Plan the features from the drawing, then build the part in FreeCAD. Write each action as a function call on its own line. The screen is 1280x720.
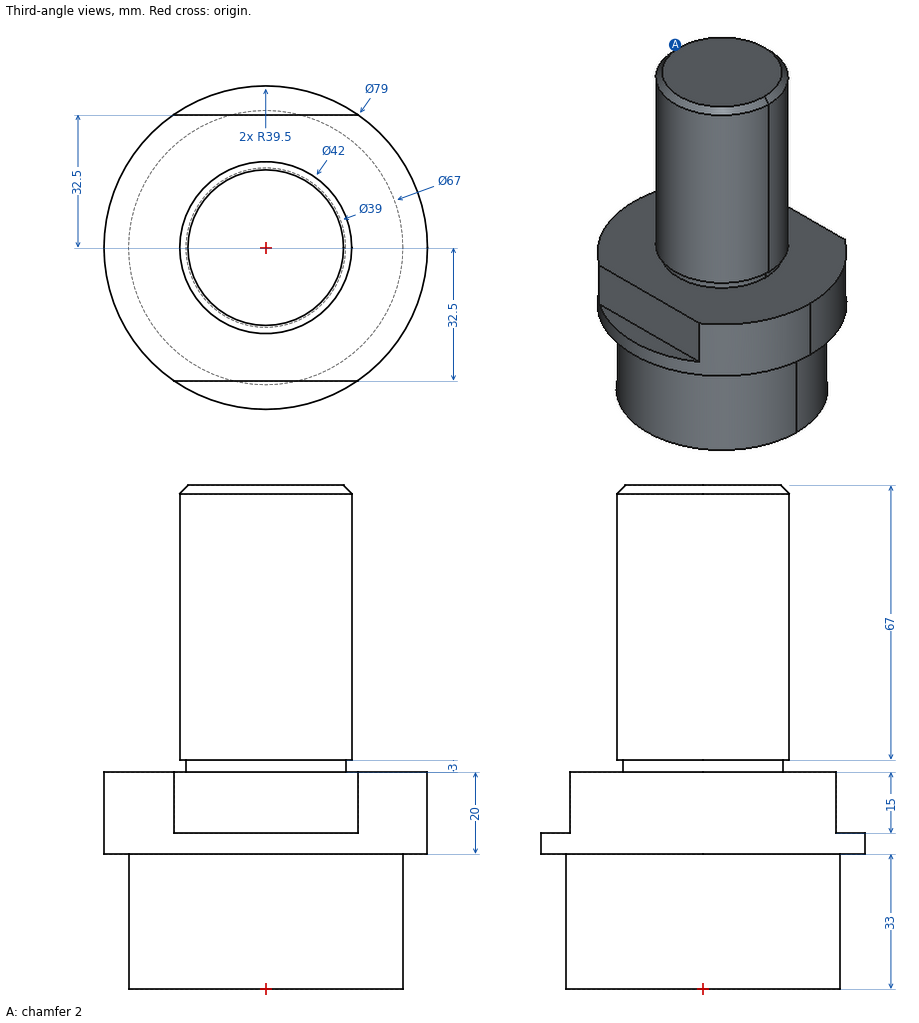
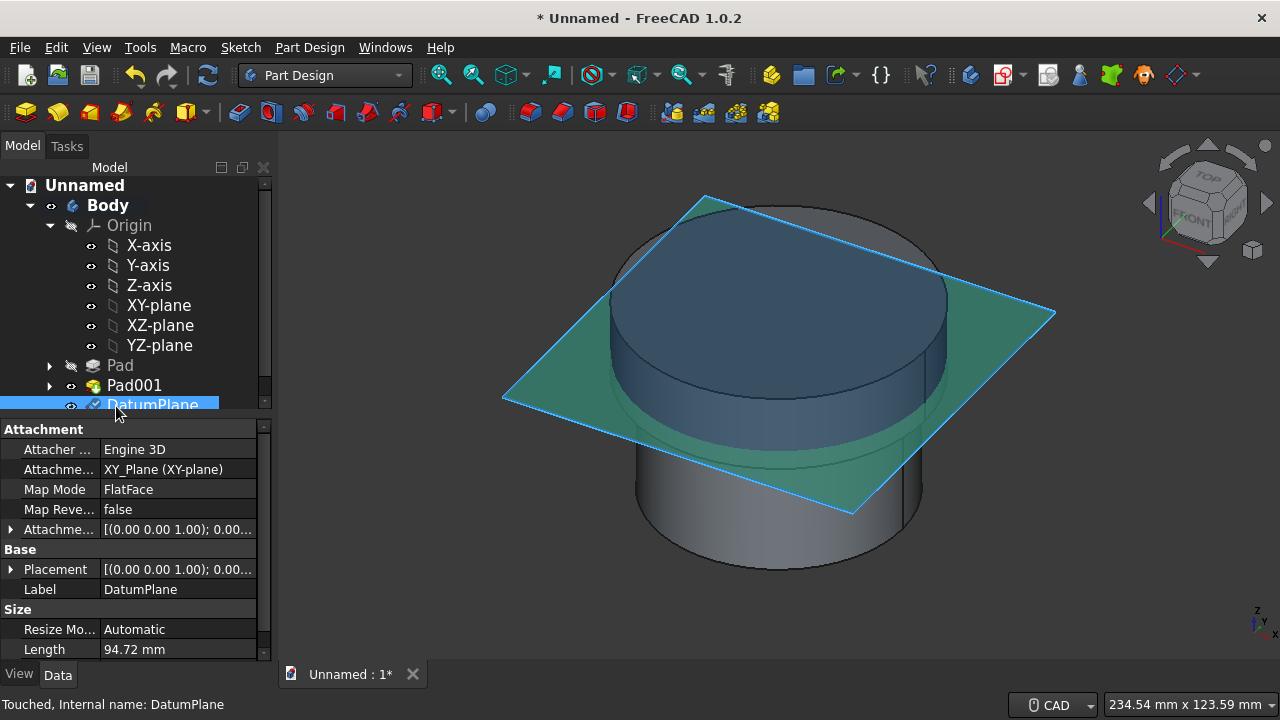
click(1004, 76)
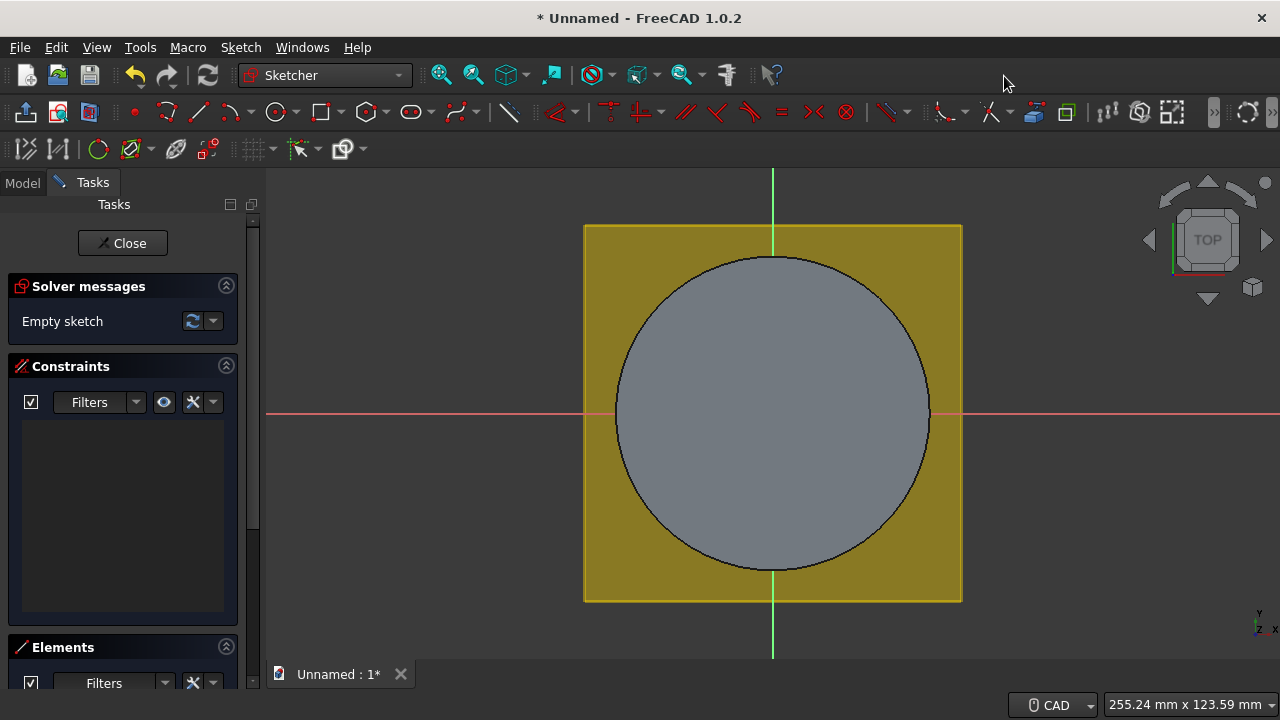
click(90, 112)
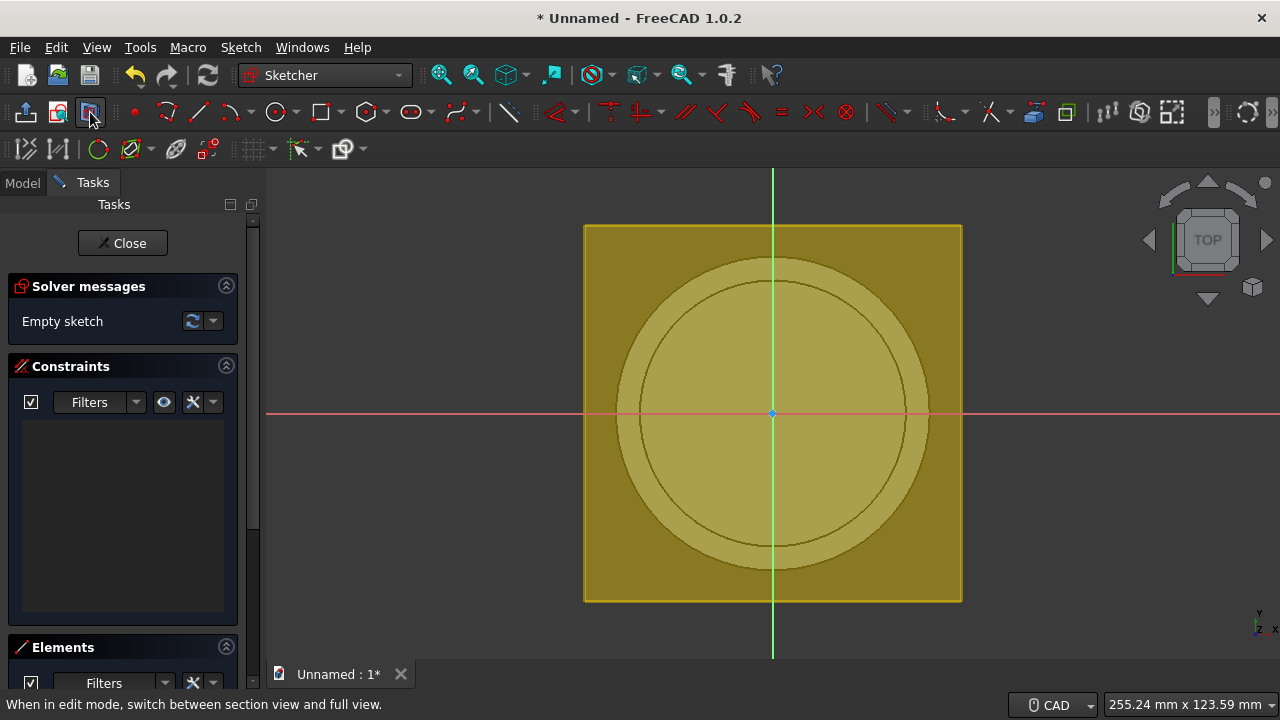
click(200, 112)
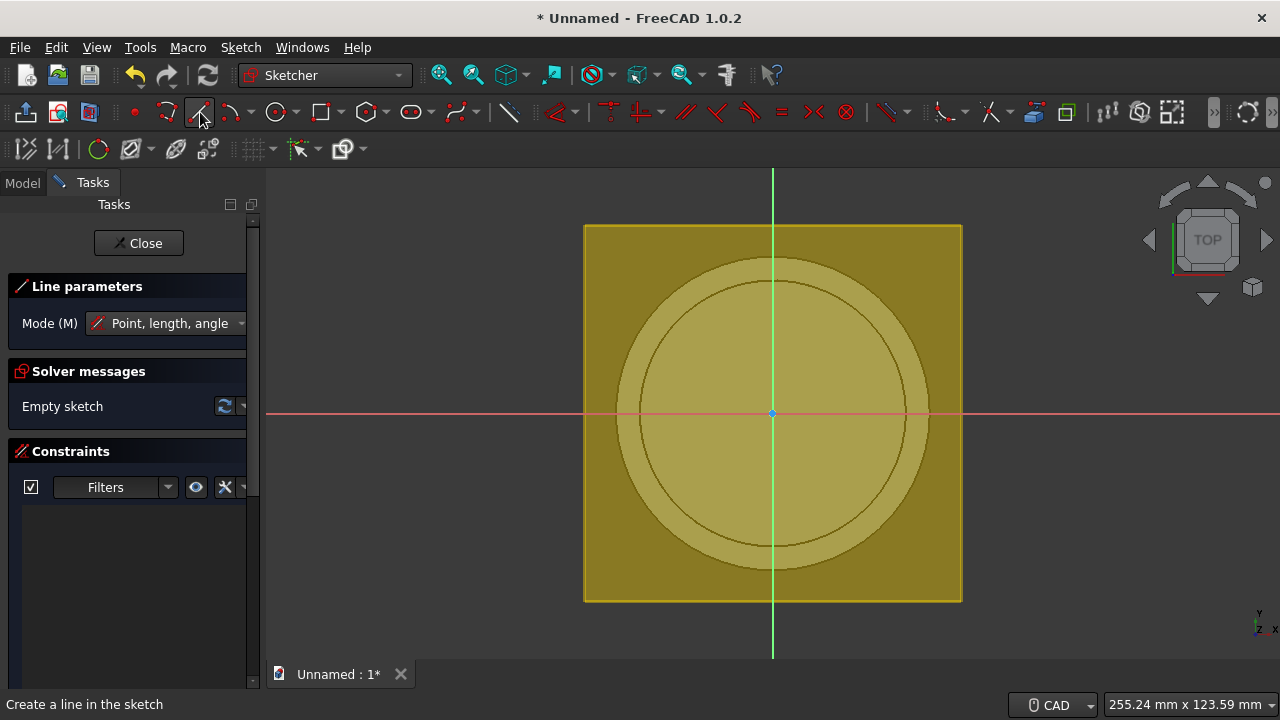
click(684, 284)
click(862, 284)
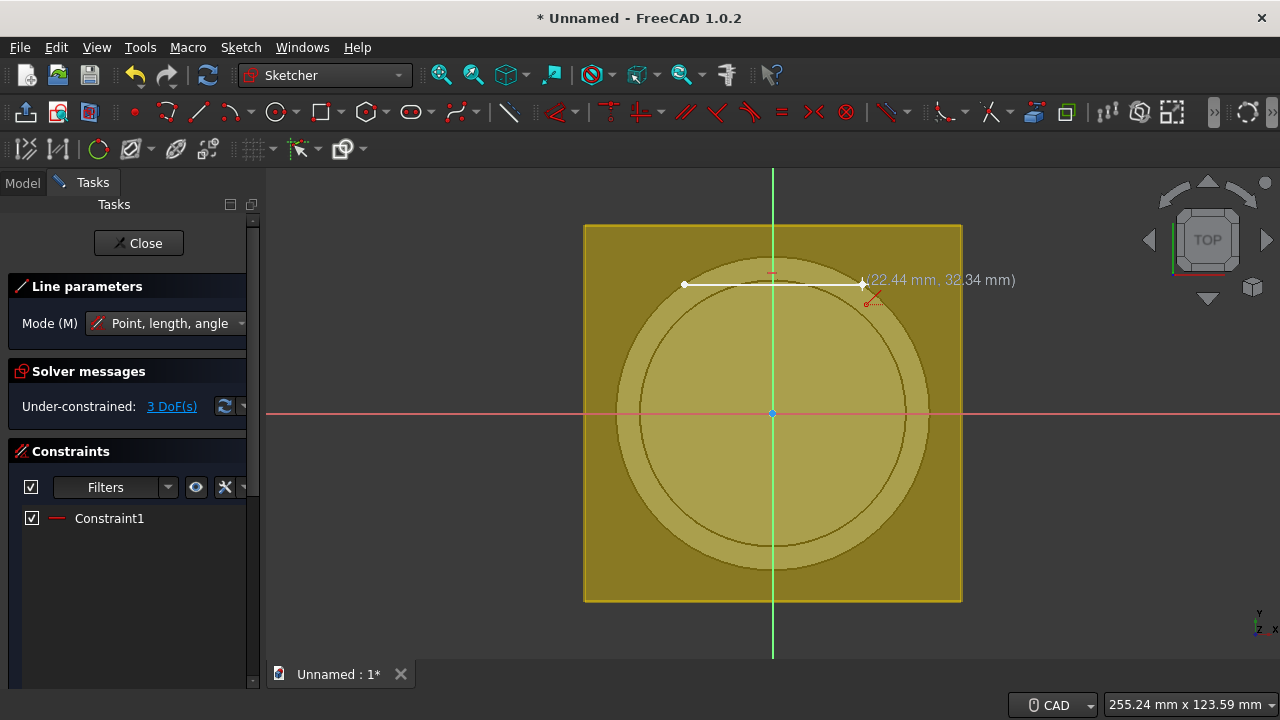
click(254, 112)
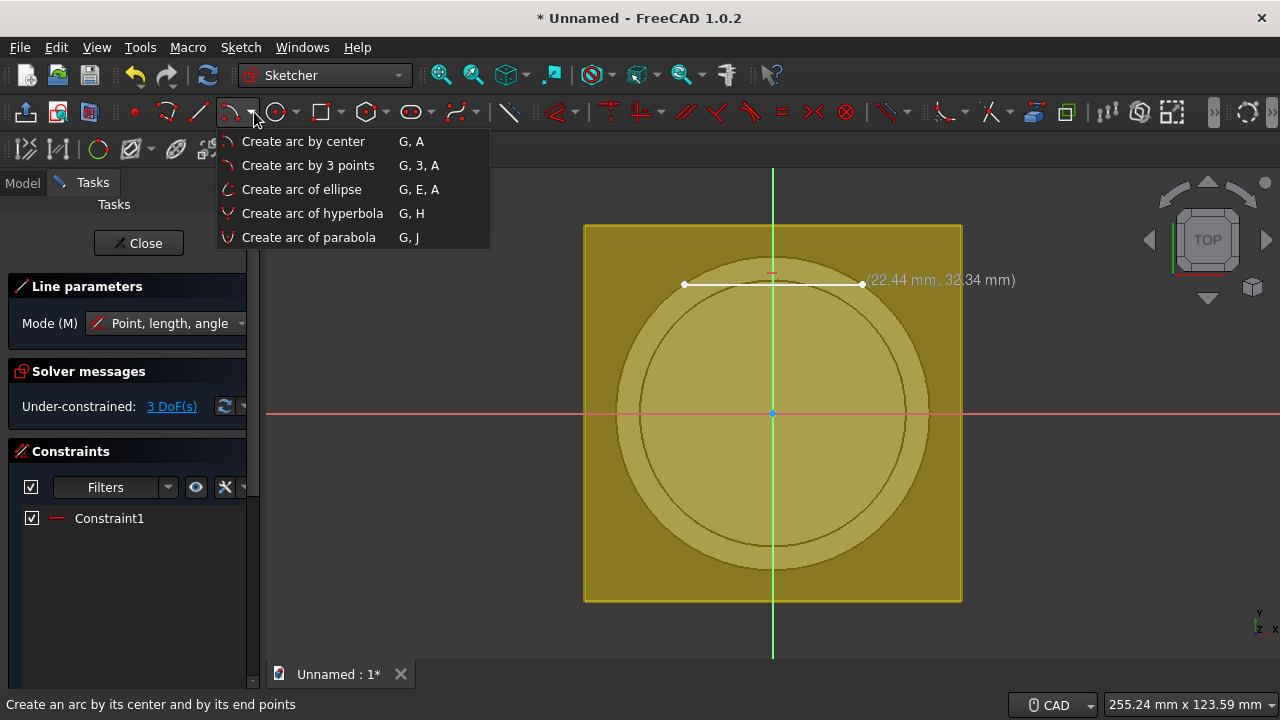
click(354, 165)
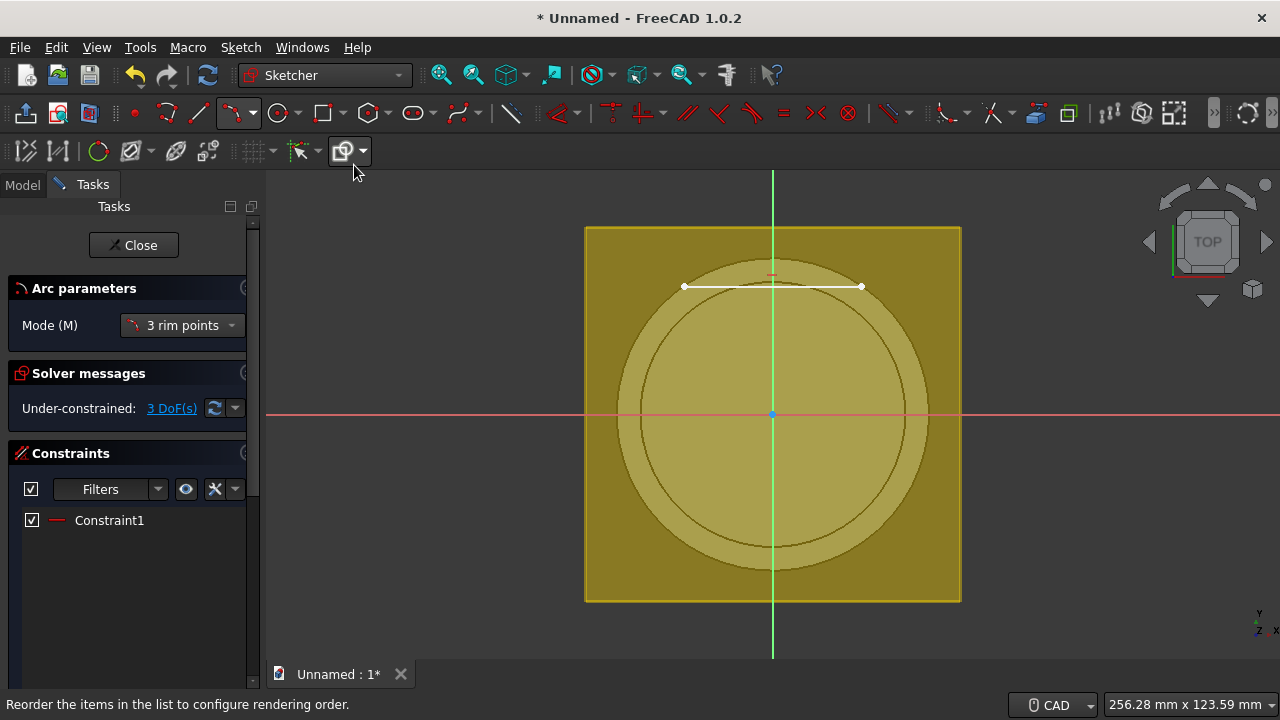
click(862, 287)
click(684, 287)
click(792, 259)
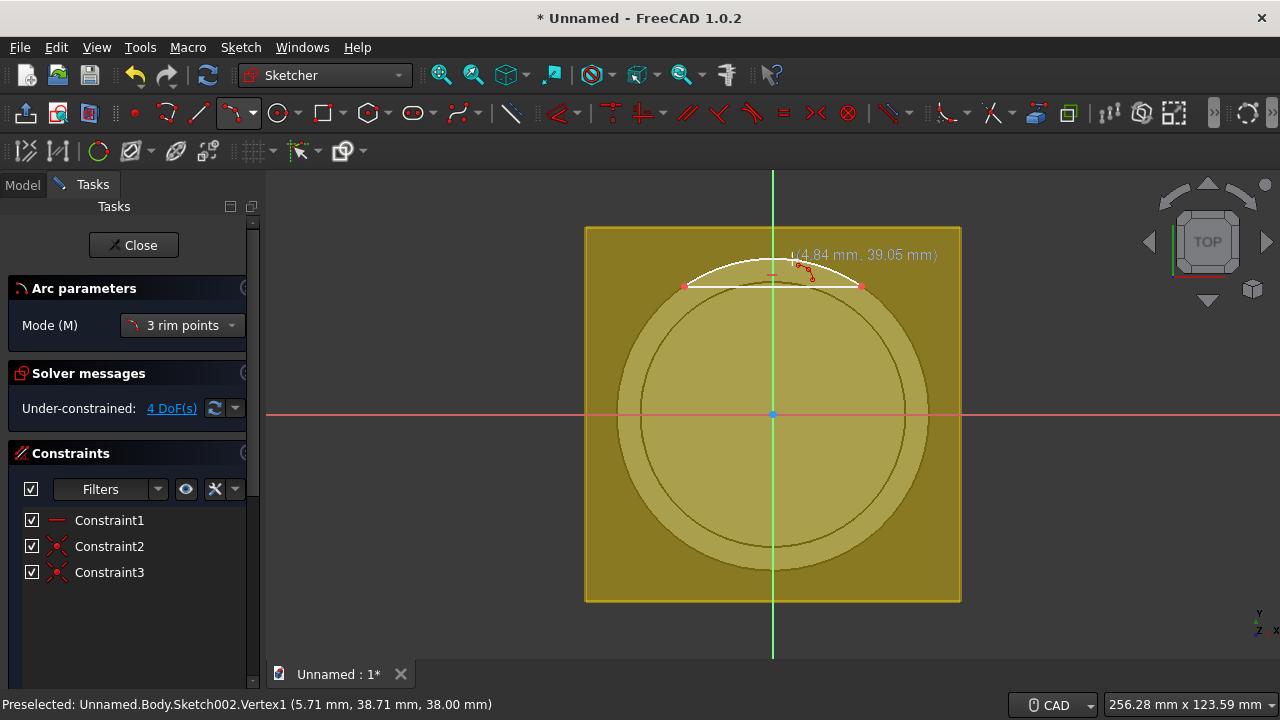
click(200, 114)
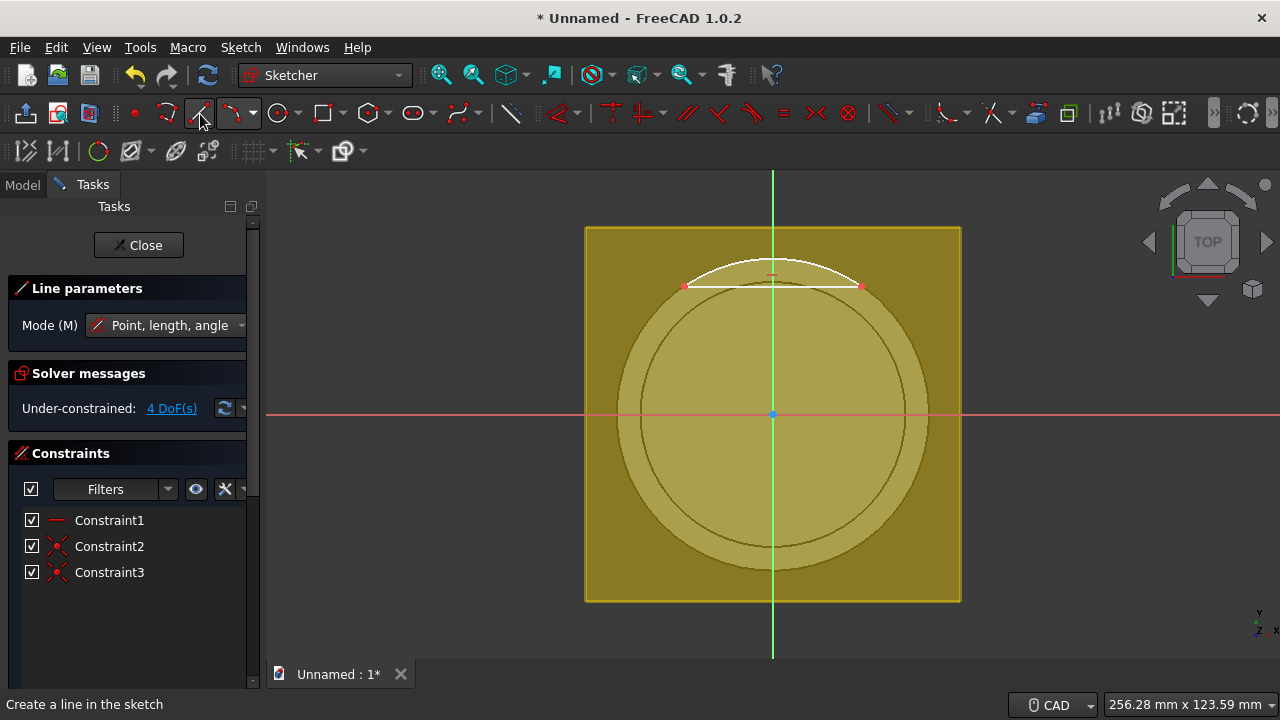
click(862, 543)
click(684, 543)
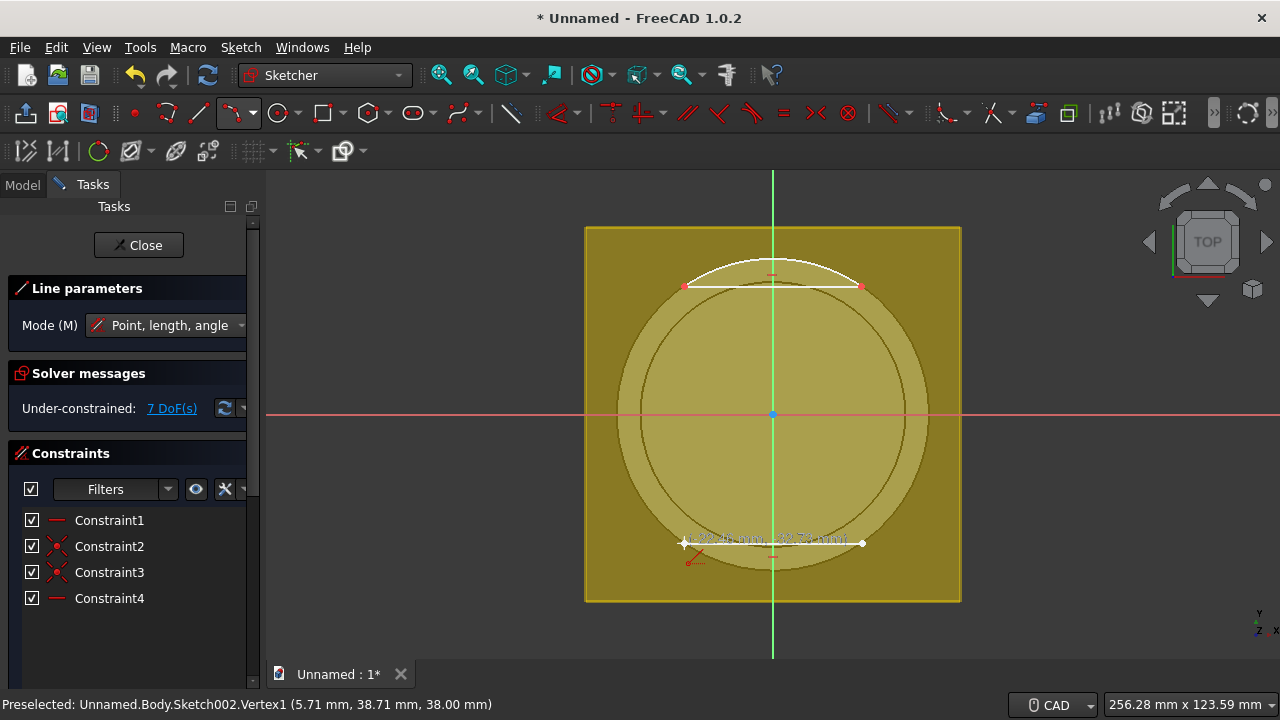
click(232, 114)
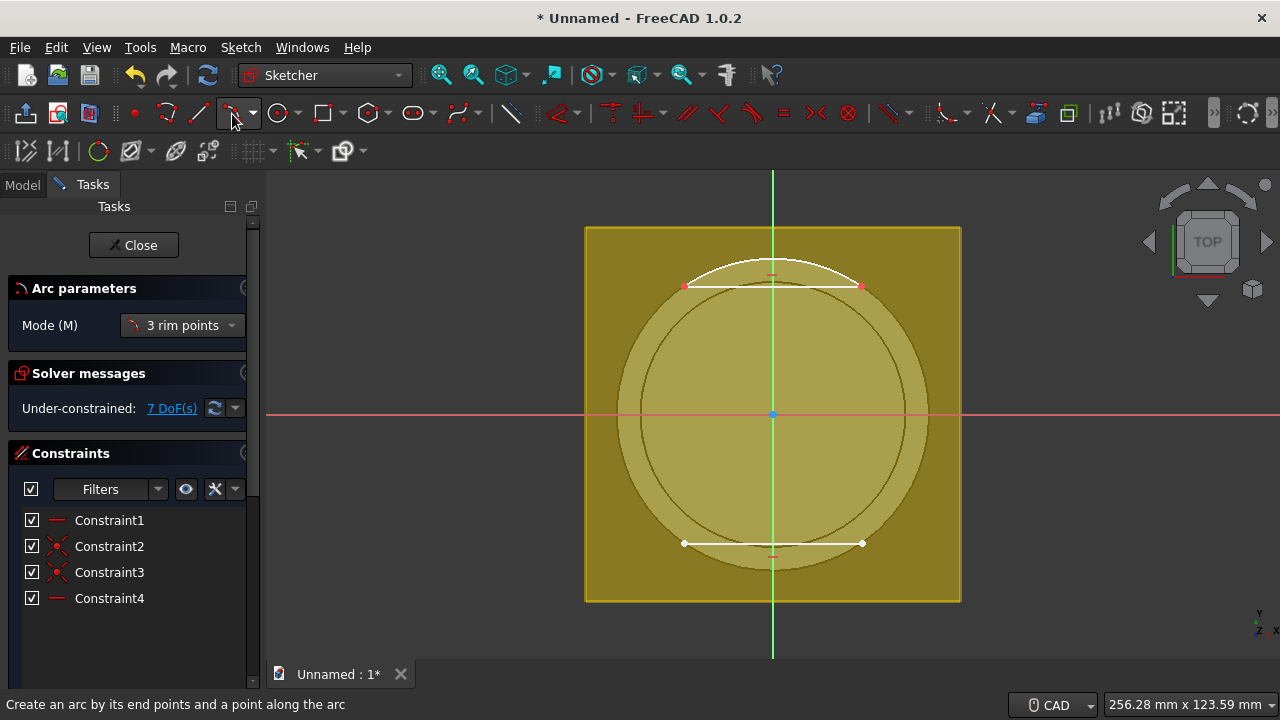
click(684, 544)
click(862, 544)
click(754, 570)
key(Escape)